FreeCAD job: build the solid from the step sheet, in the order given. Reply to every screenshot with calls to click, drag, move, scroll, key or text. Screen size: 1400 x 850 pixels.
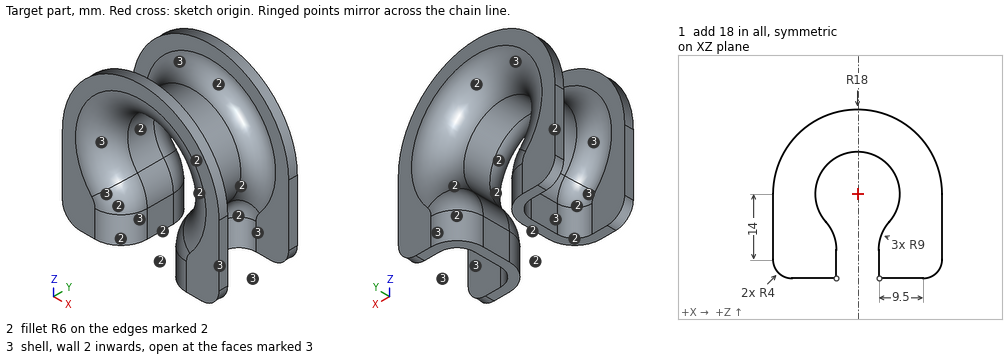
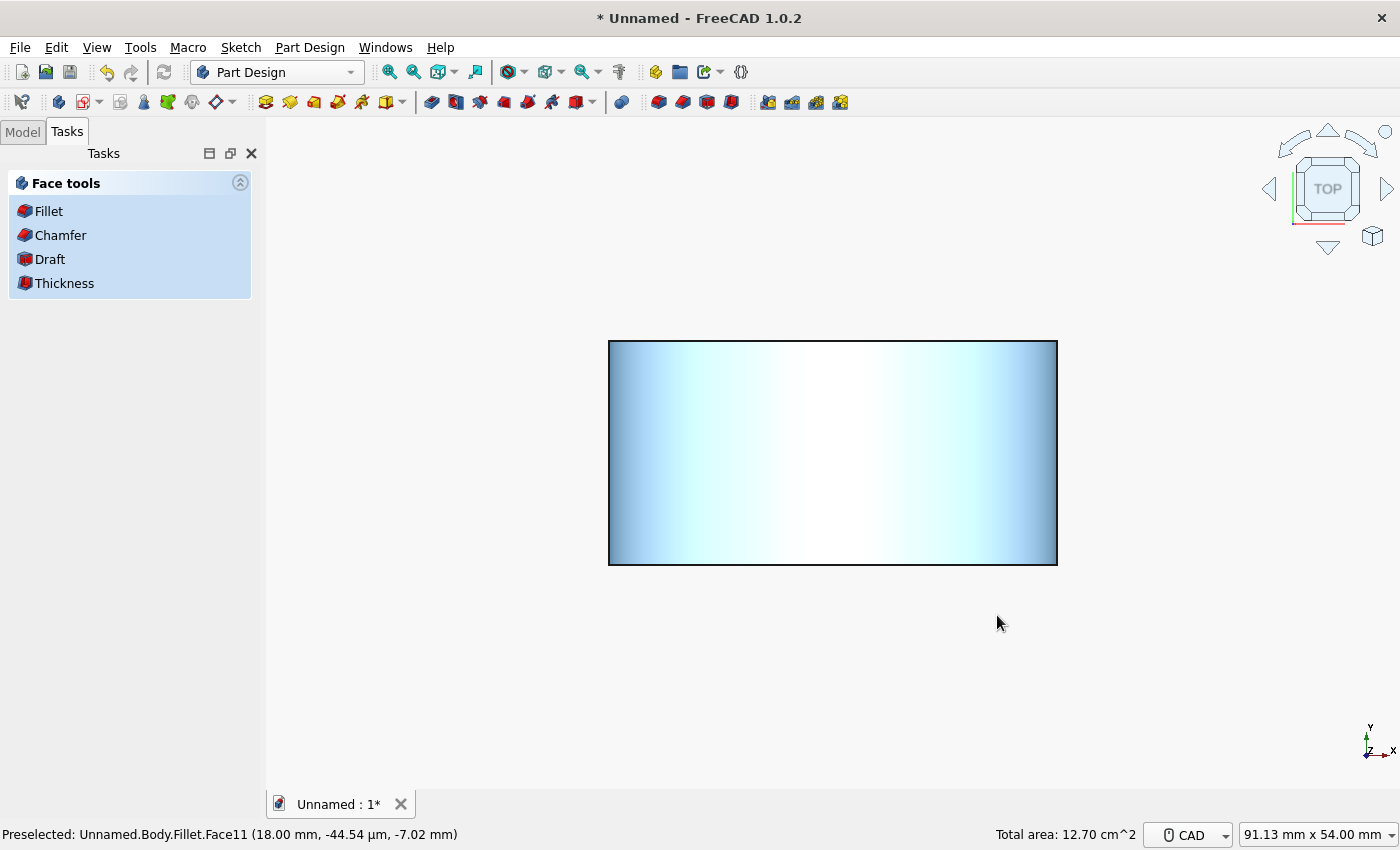
key(v)
key(f)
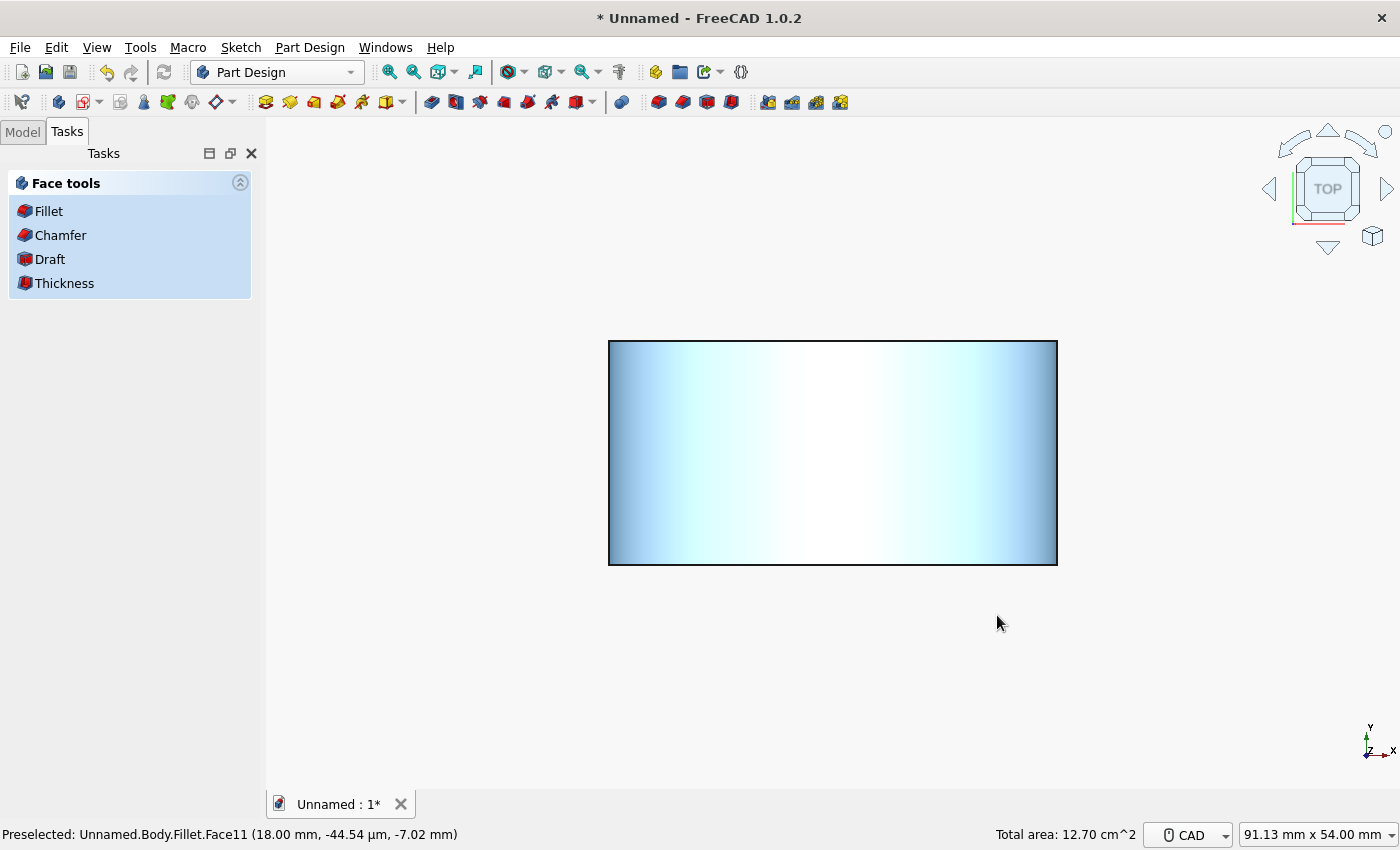
key(0)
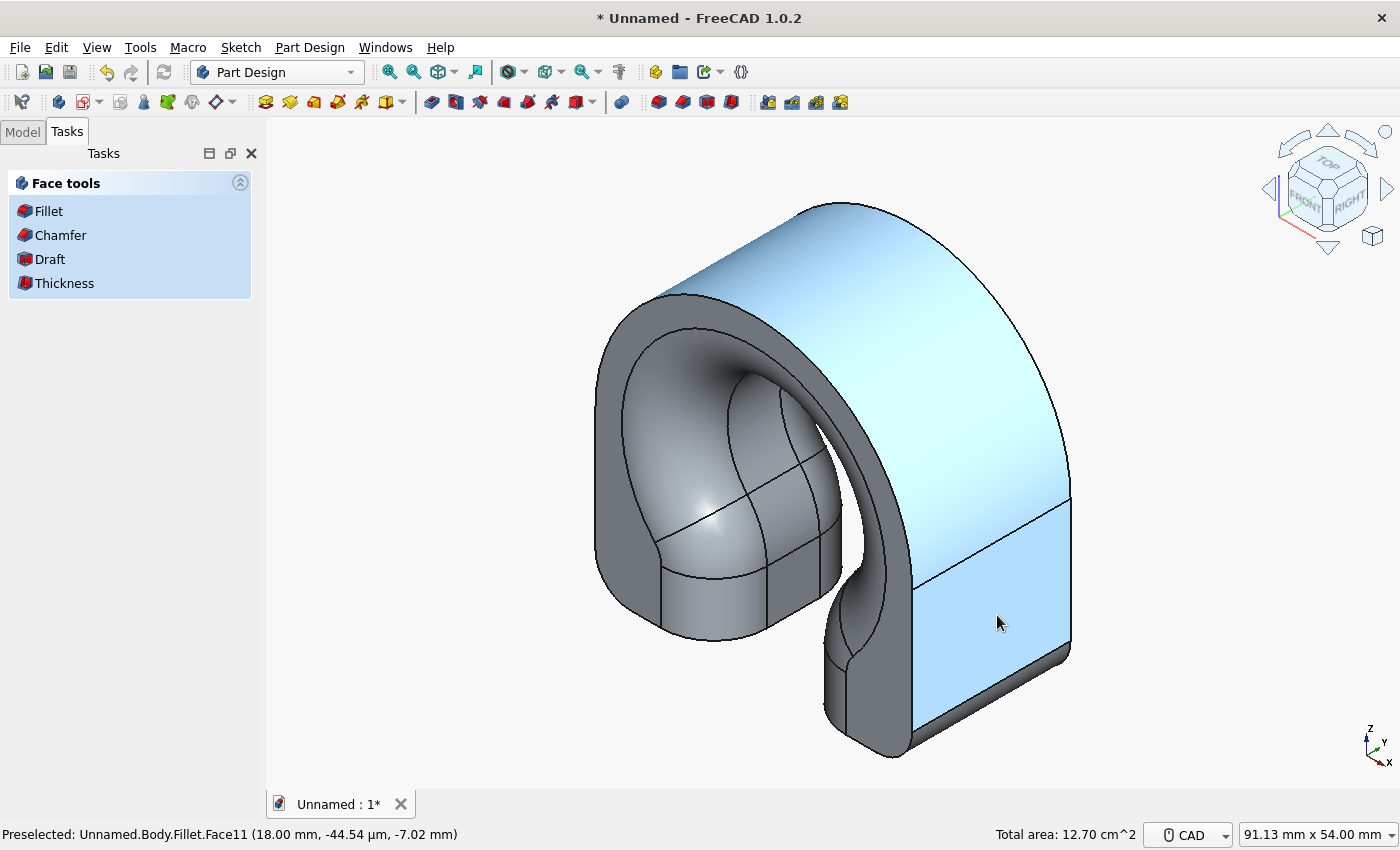
key(1)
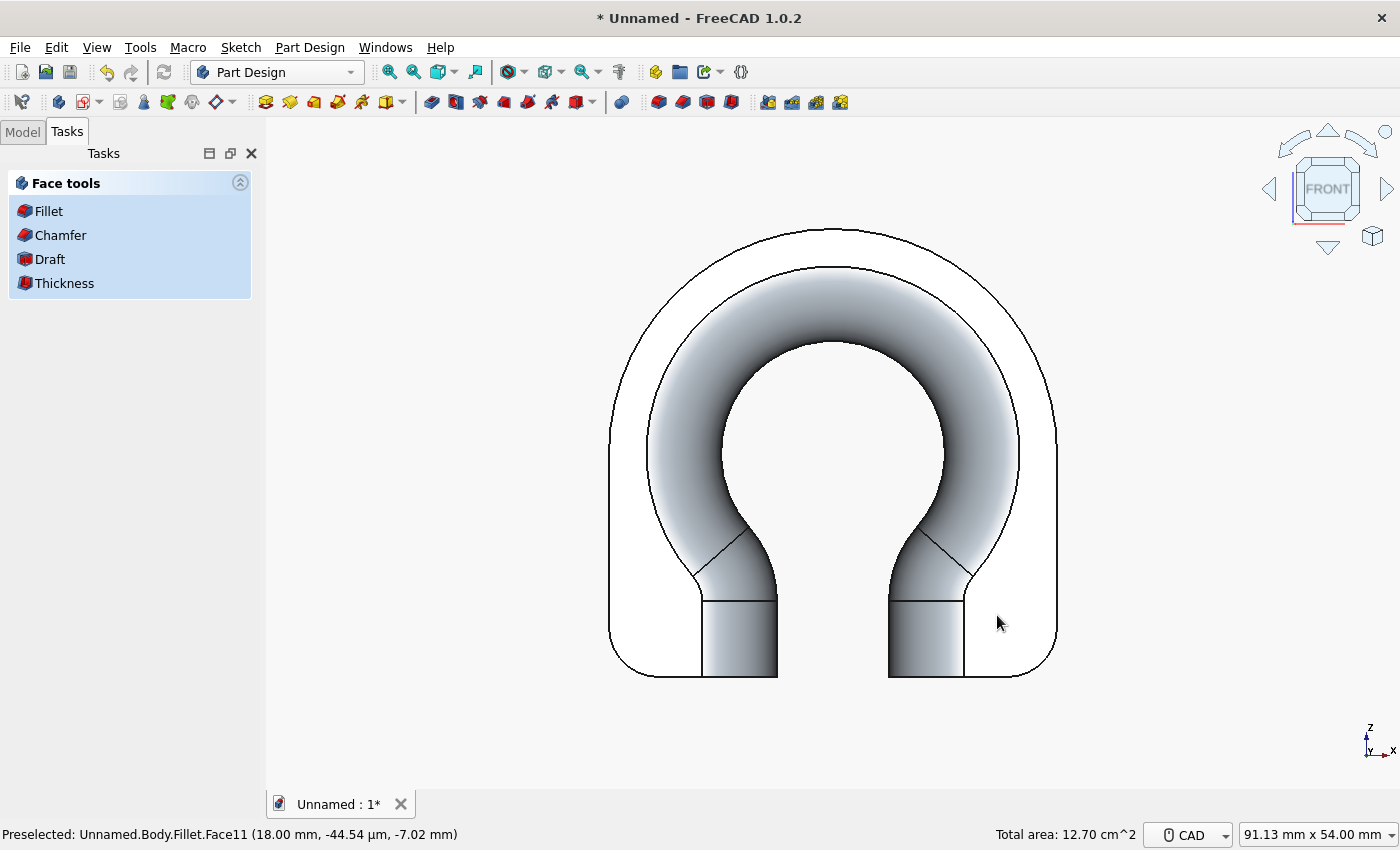
key(3)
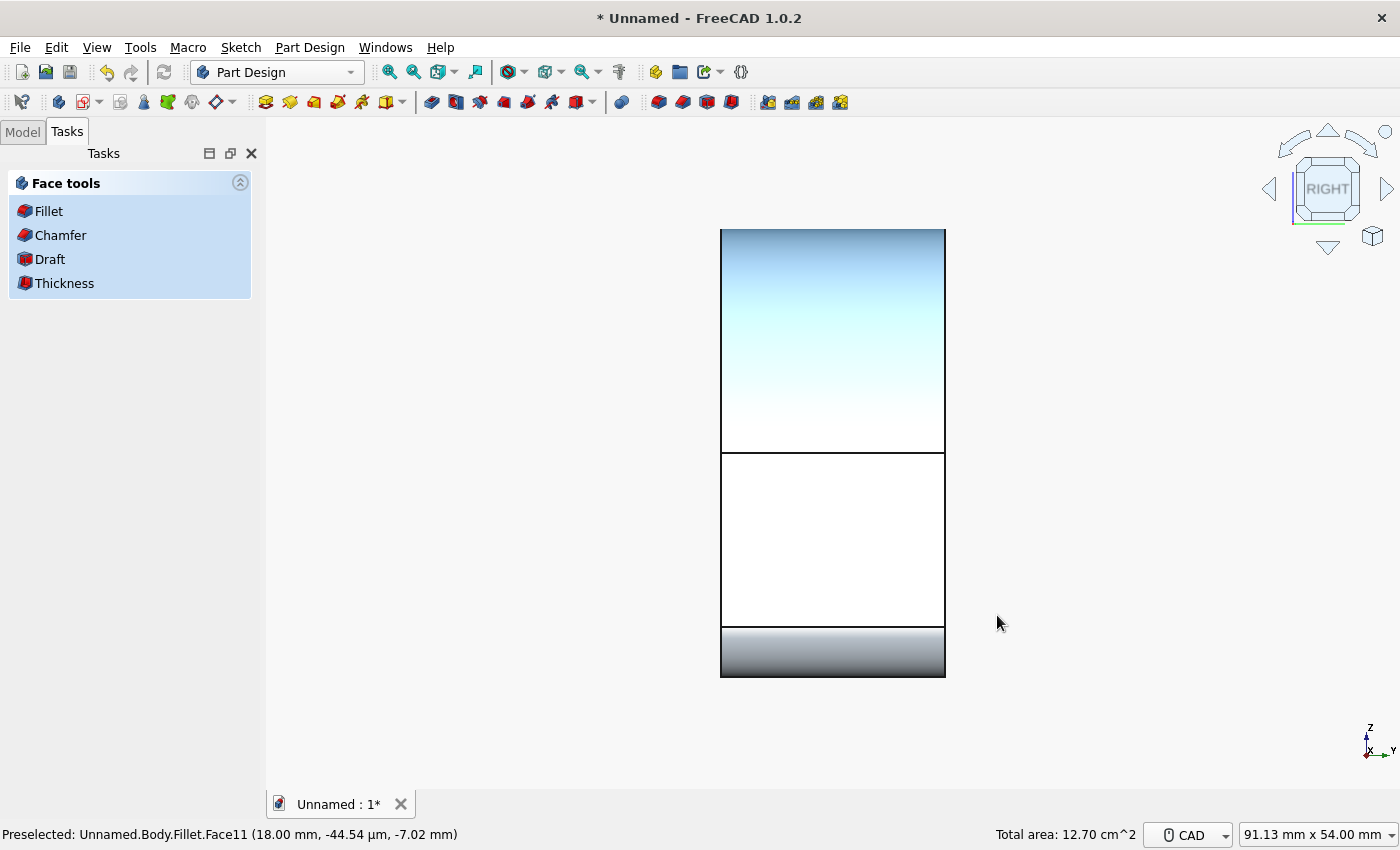
click(897, 661, ctrl)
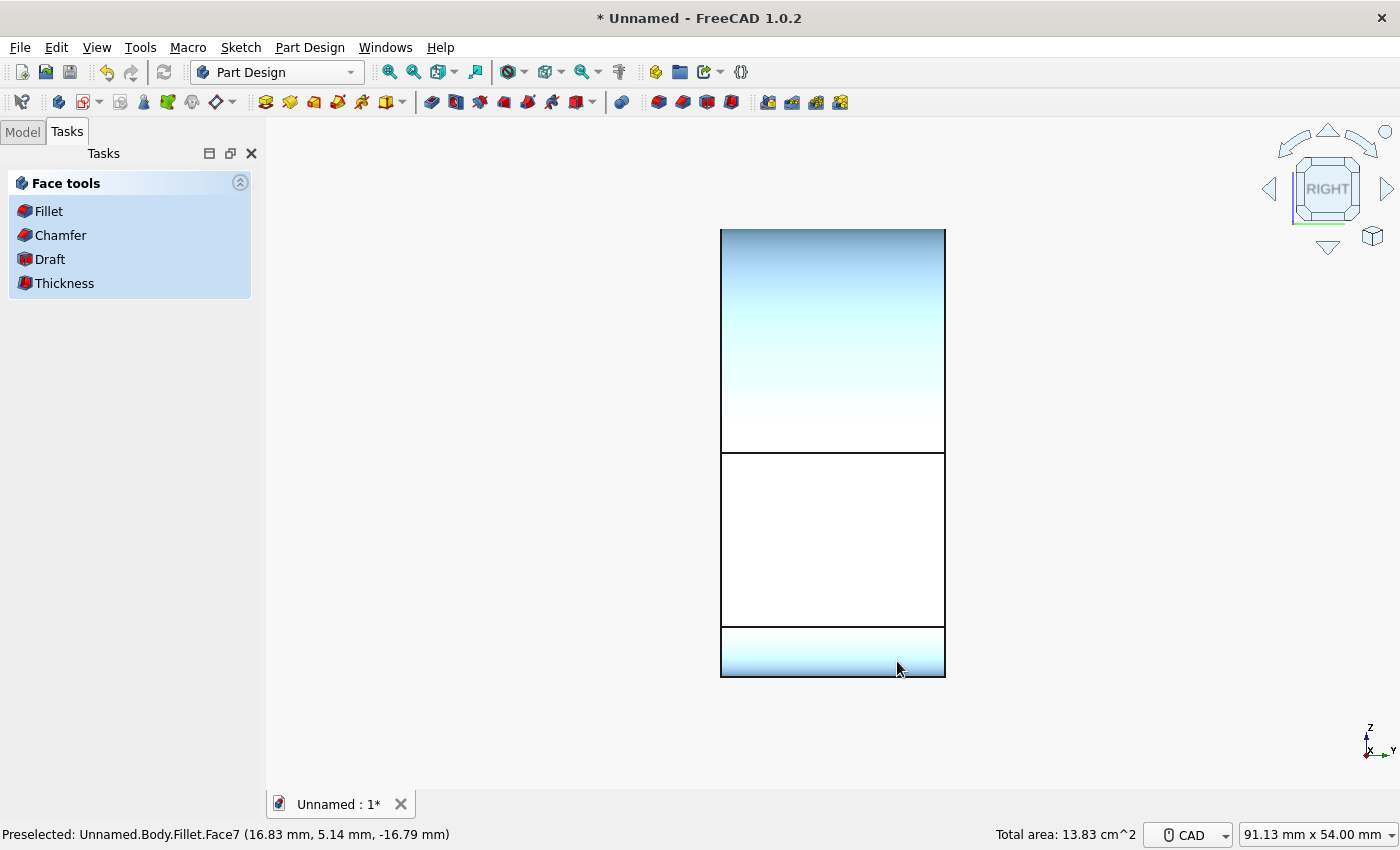
key(5)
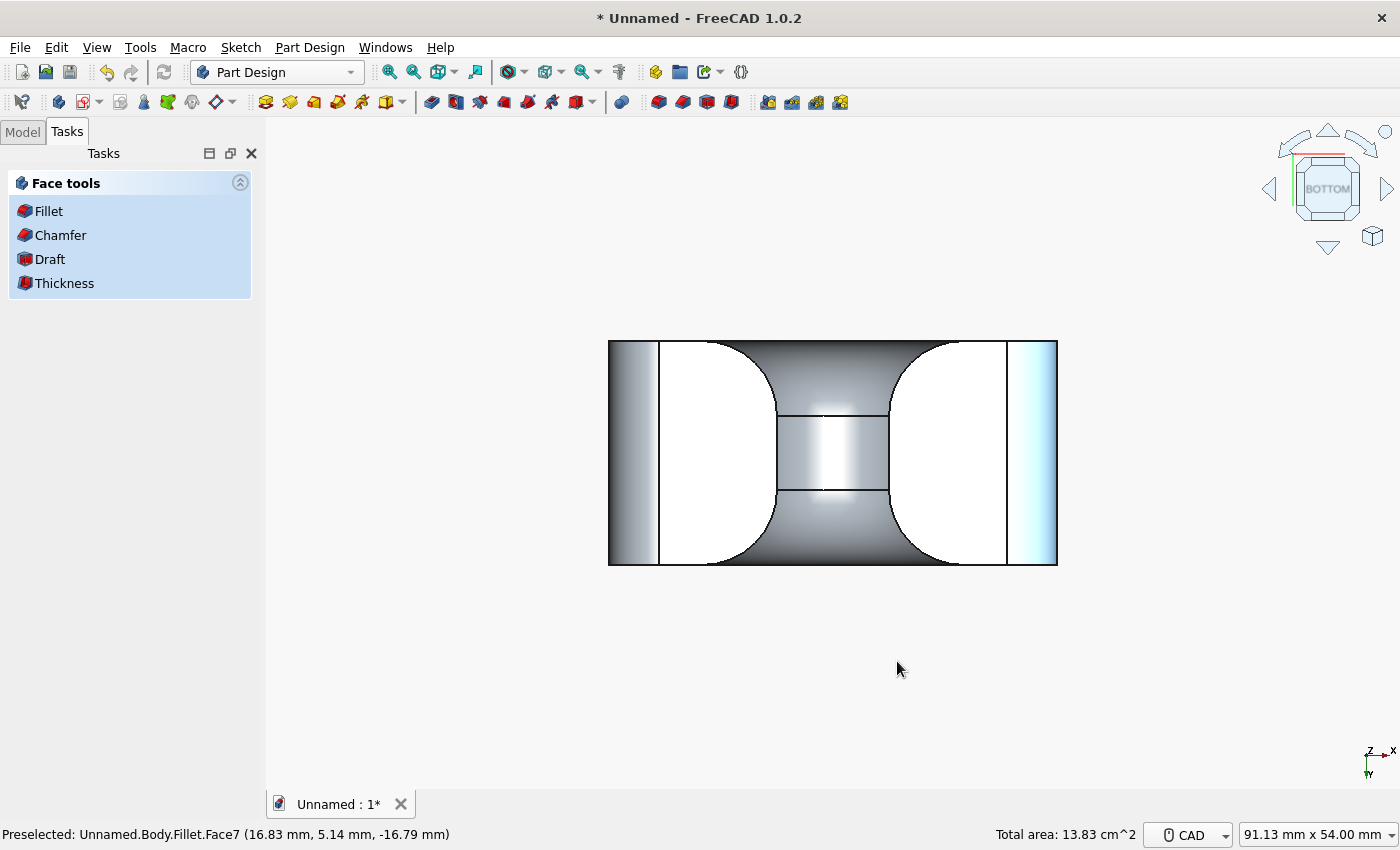
click(390, 72)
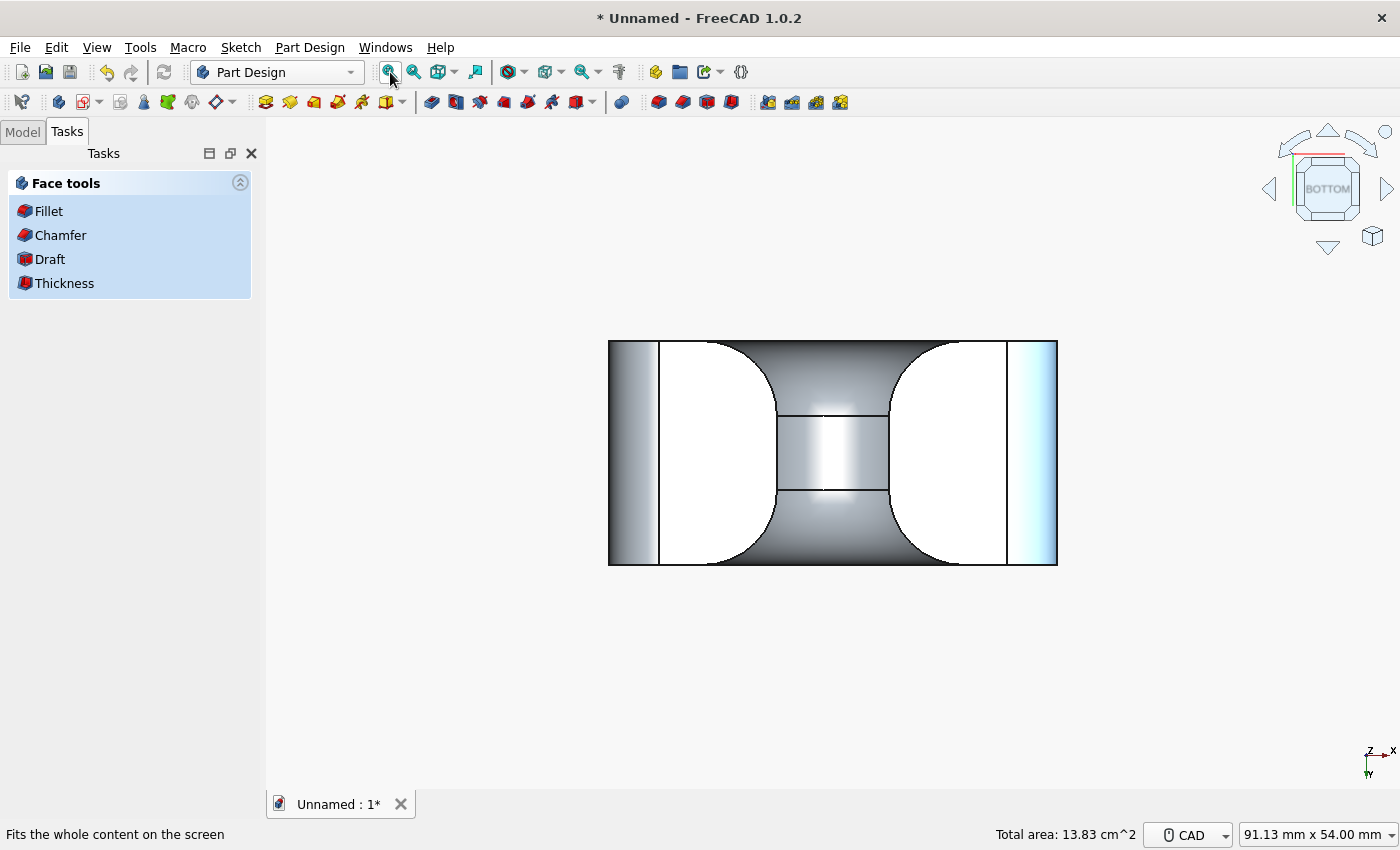
click(718, 484, ctrl)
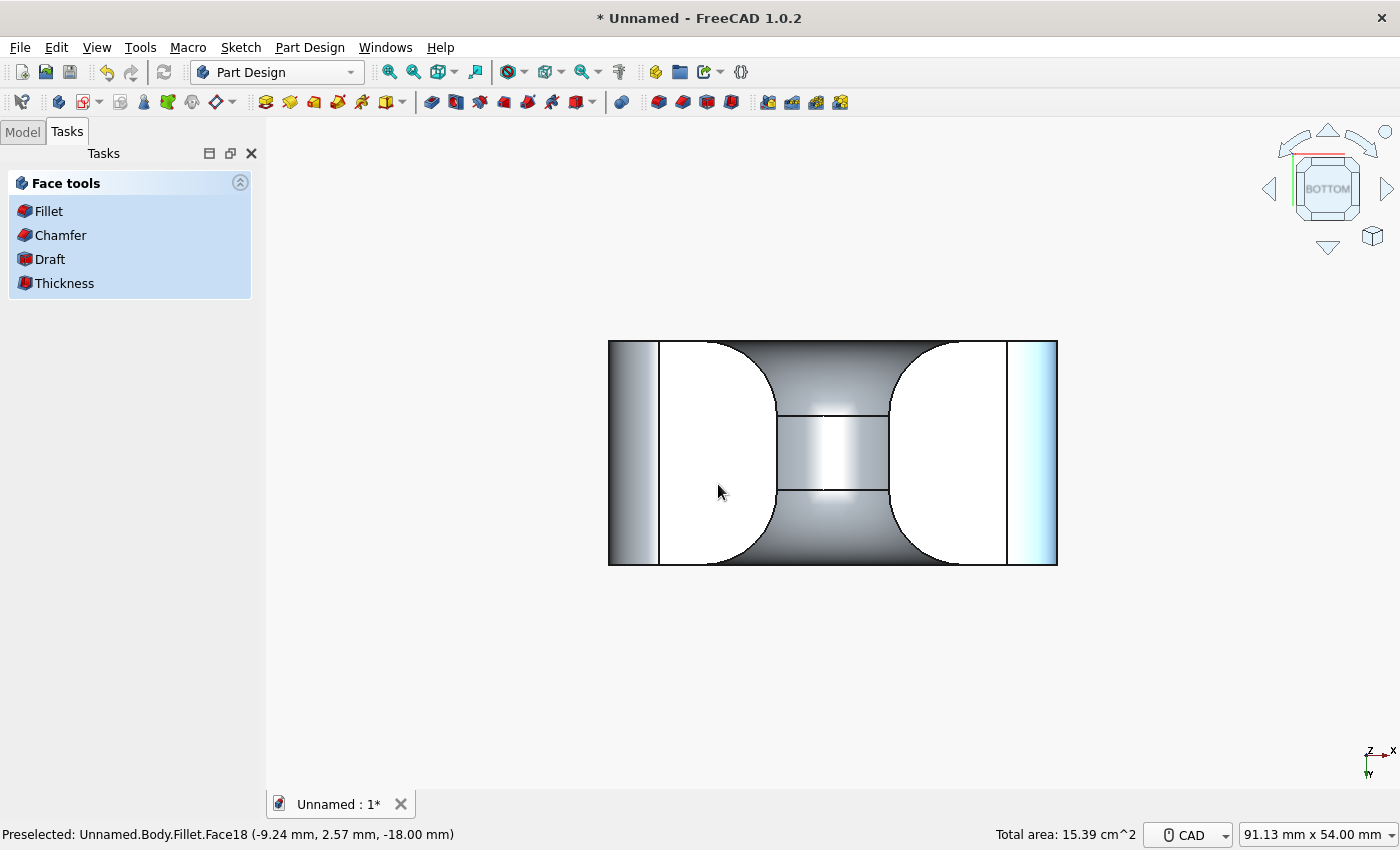
click(624, 484, ctrl)